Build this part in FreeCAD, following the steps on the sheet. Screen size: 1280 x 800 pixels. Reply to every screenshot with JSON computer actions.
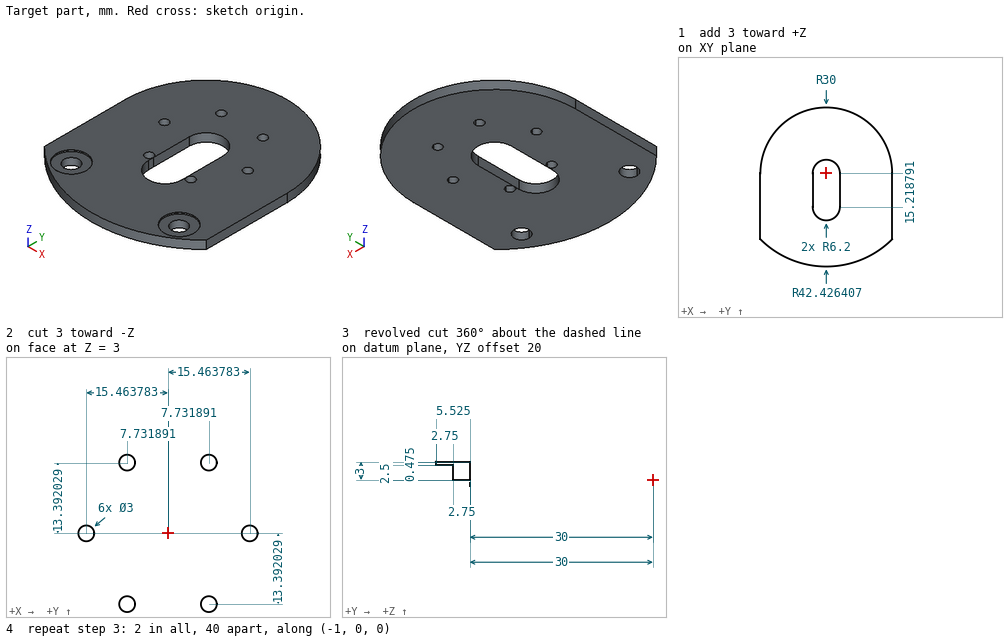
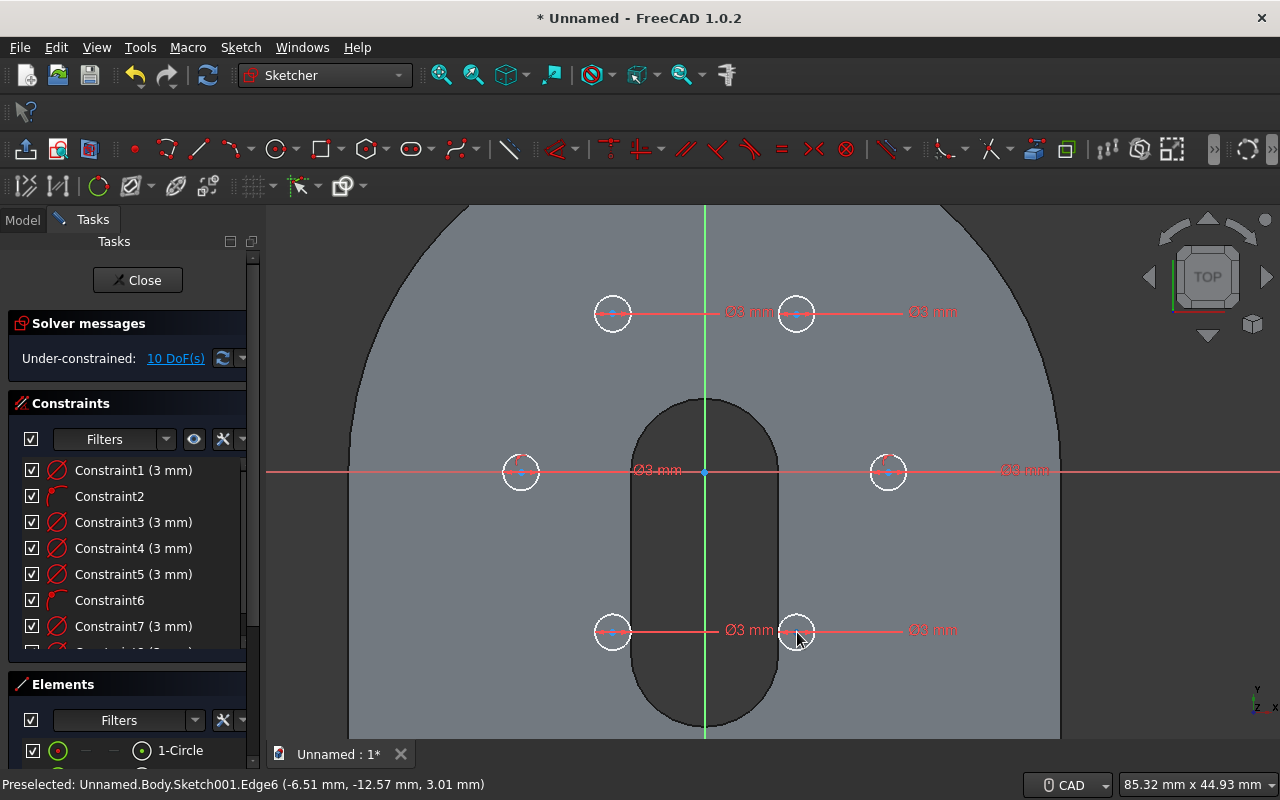
{"action": "left_click", "coordinate": [613, 314]}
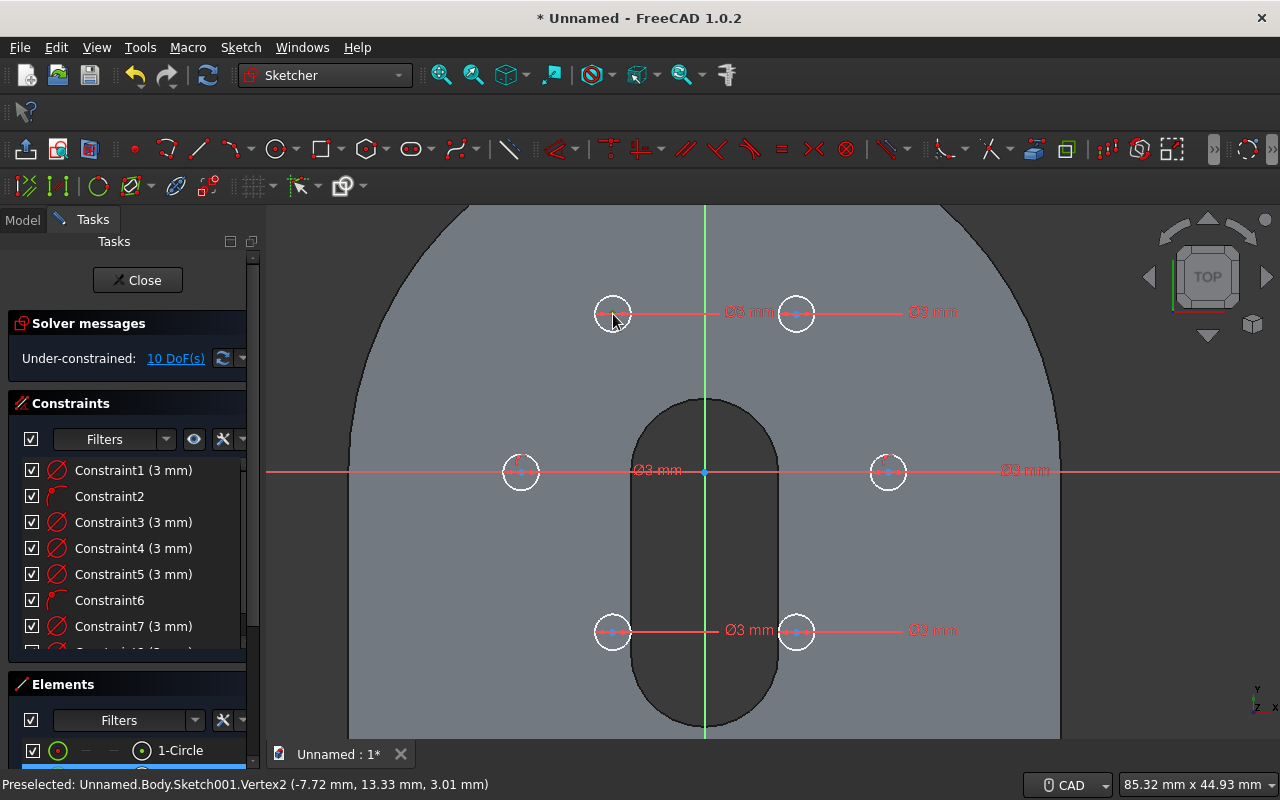
{"action": "left_click", "coordinate": [797, 314]}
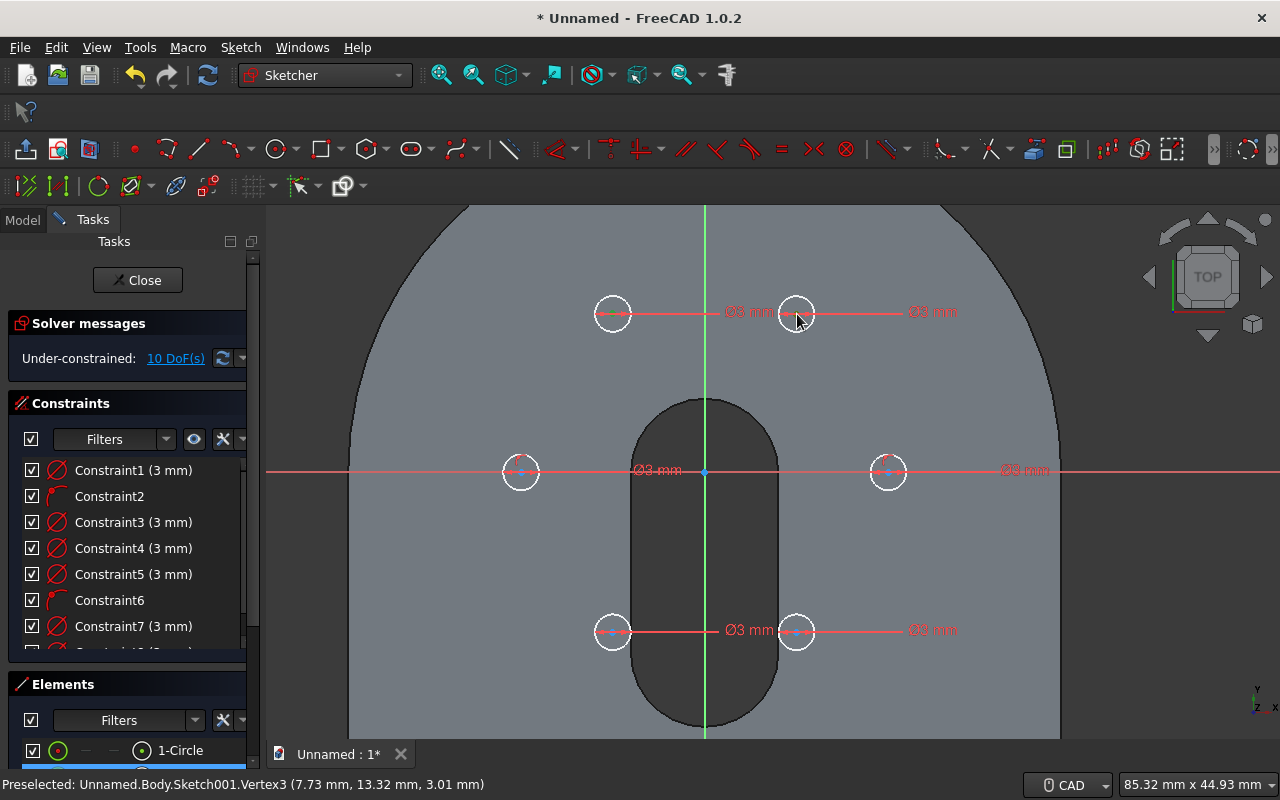
{"action": "key", "text": "h"}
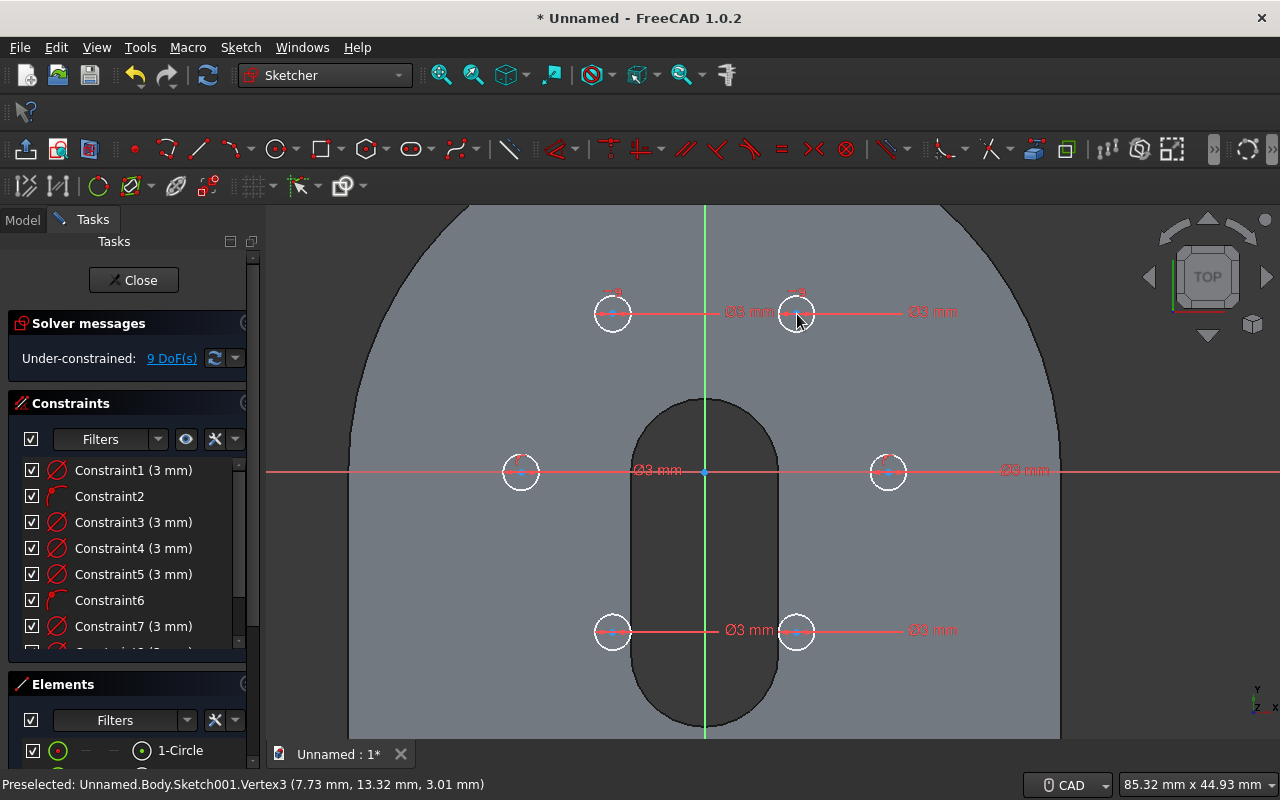
{"action": "left_click", "coordinate": [797, 314]}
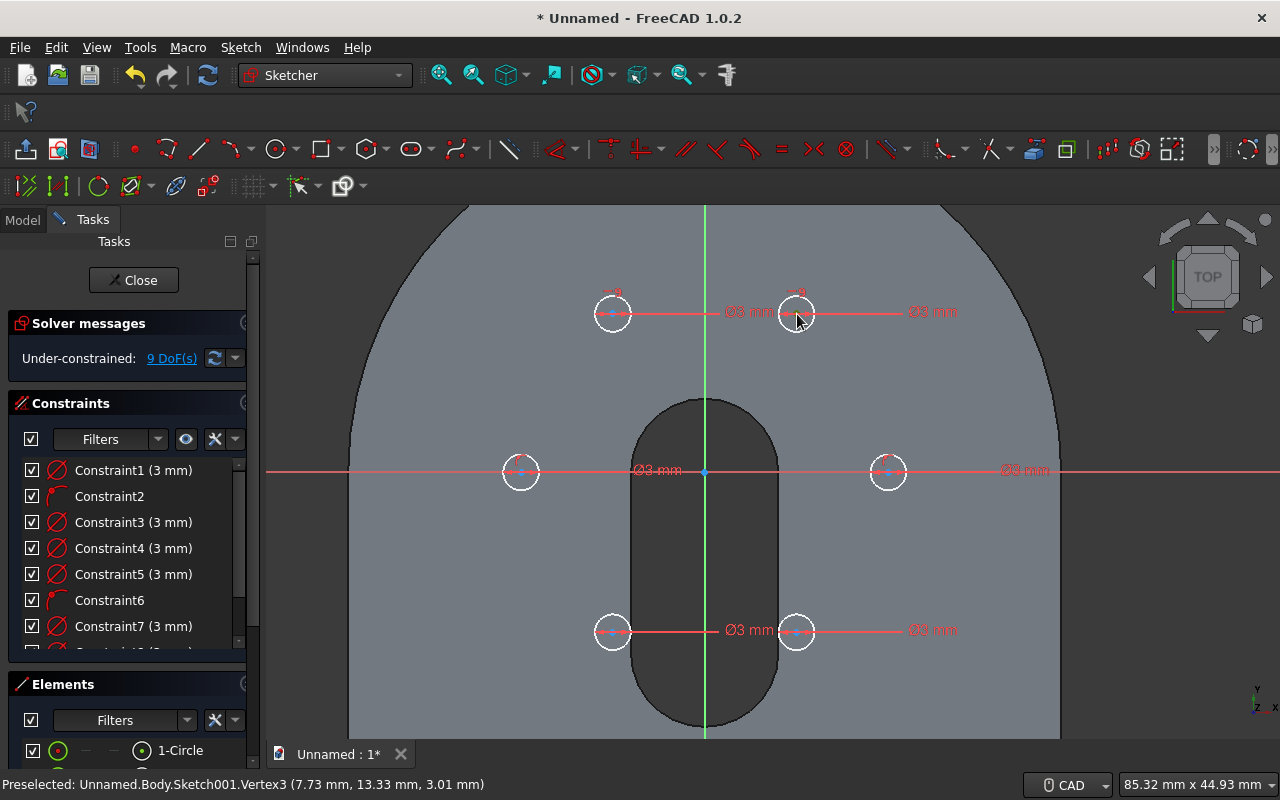
{"action": "left_click", "coordinate": [797, 632]}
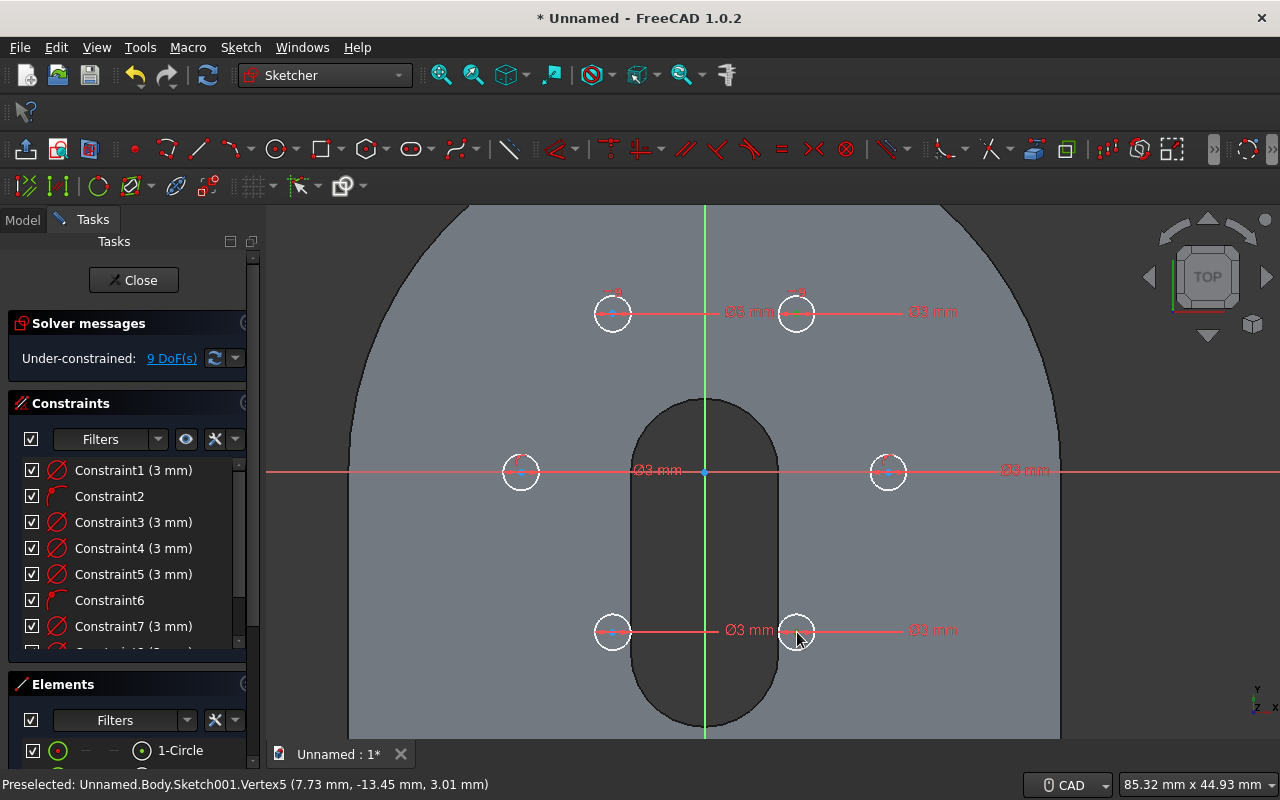
{"action": "left_click", "coordinate": [664, 150]}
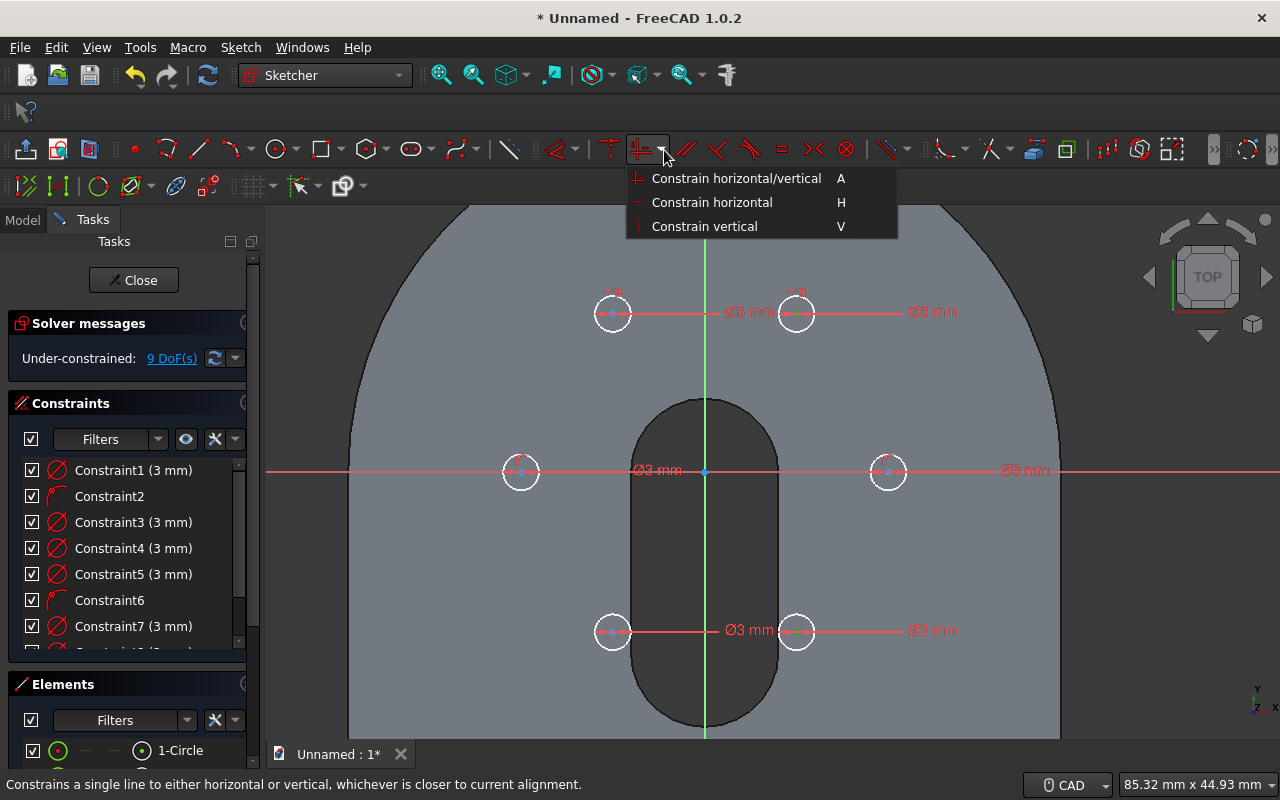
{"action": "left_click", "coordinate": [762, 226]}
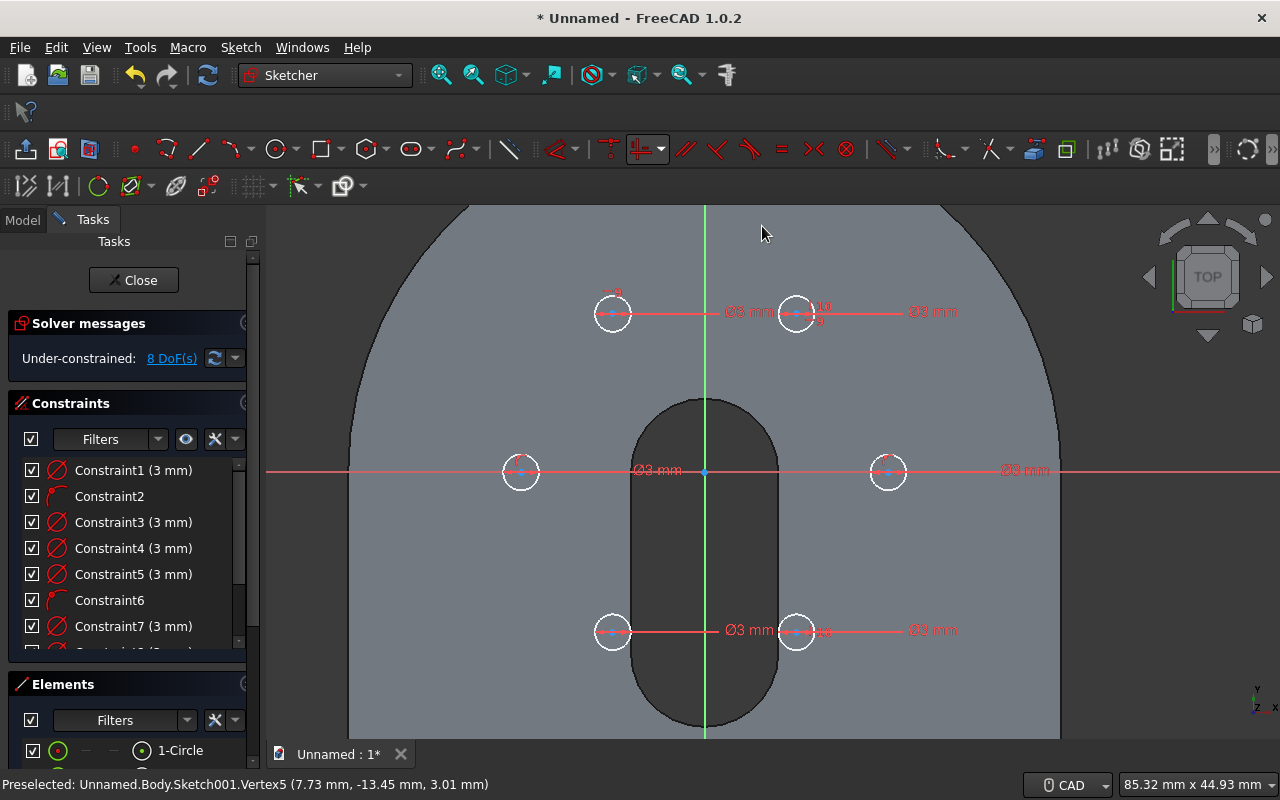
{"action": "left_click", "coordinate": [613, 314]}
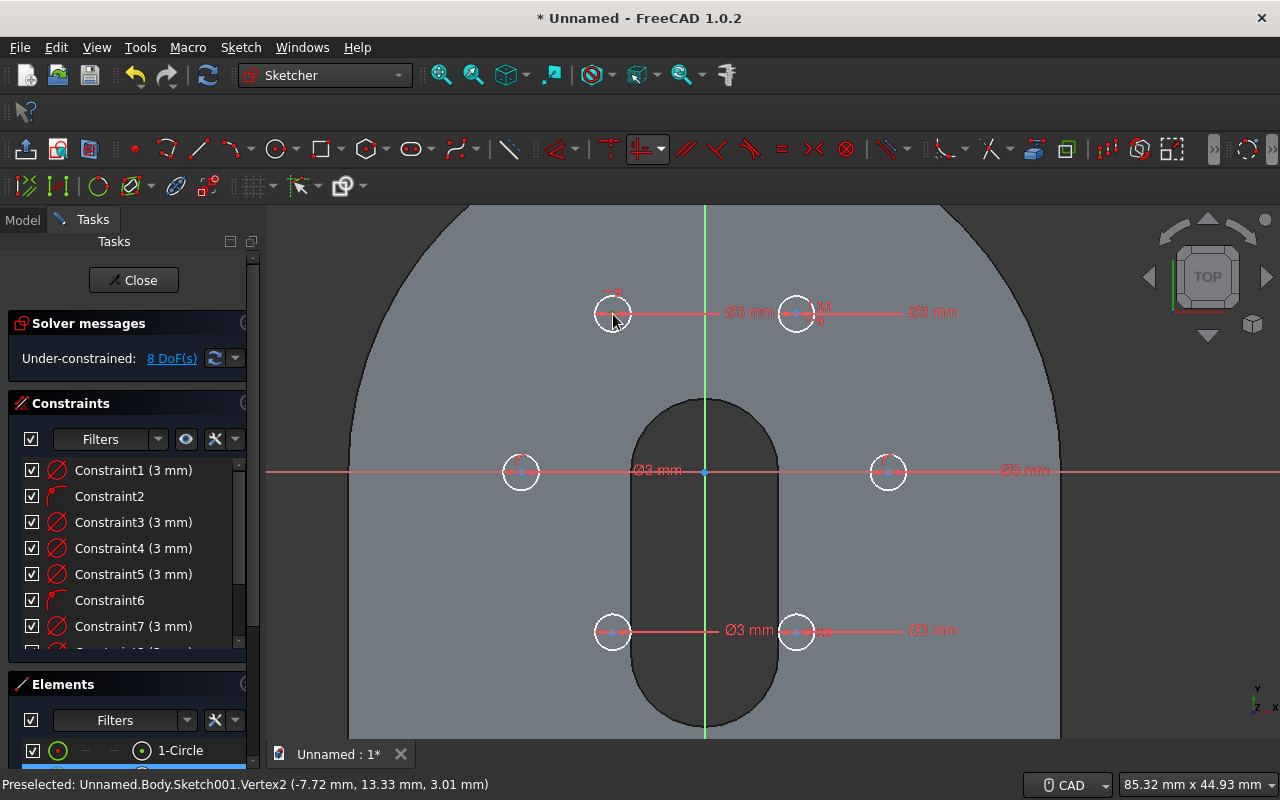
{"action": "left_click", "coordinate": [613, 632]}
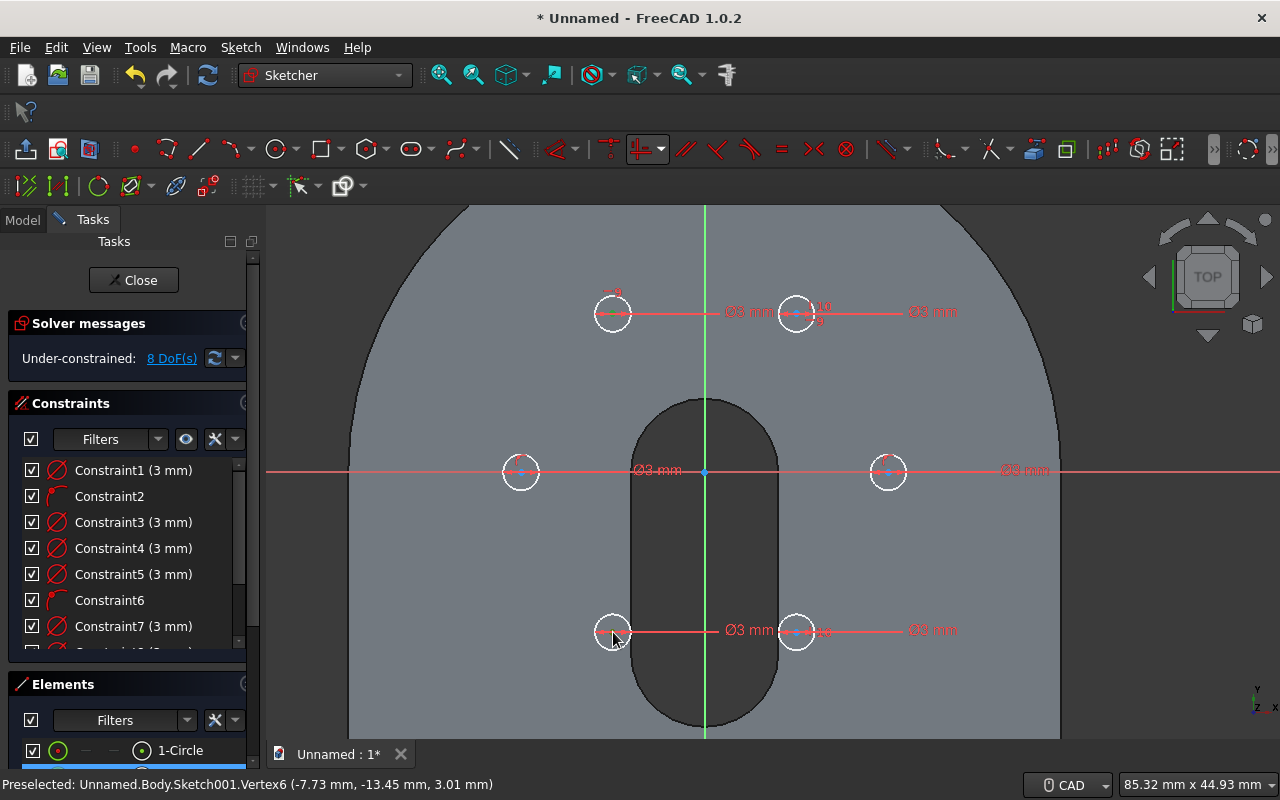
{"action": "key", "text": "v"}